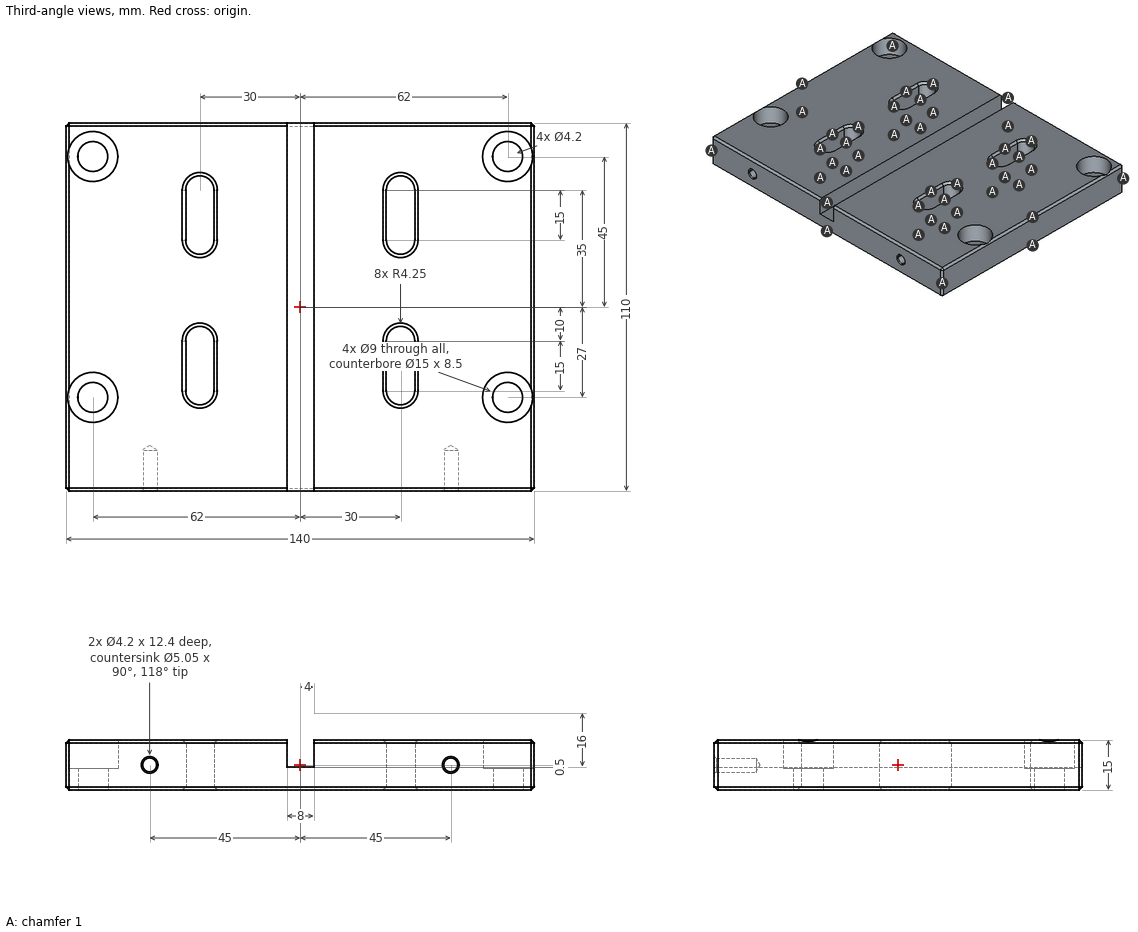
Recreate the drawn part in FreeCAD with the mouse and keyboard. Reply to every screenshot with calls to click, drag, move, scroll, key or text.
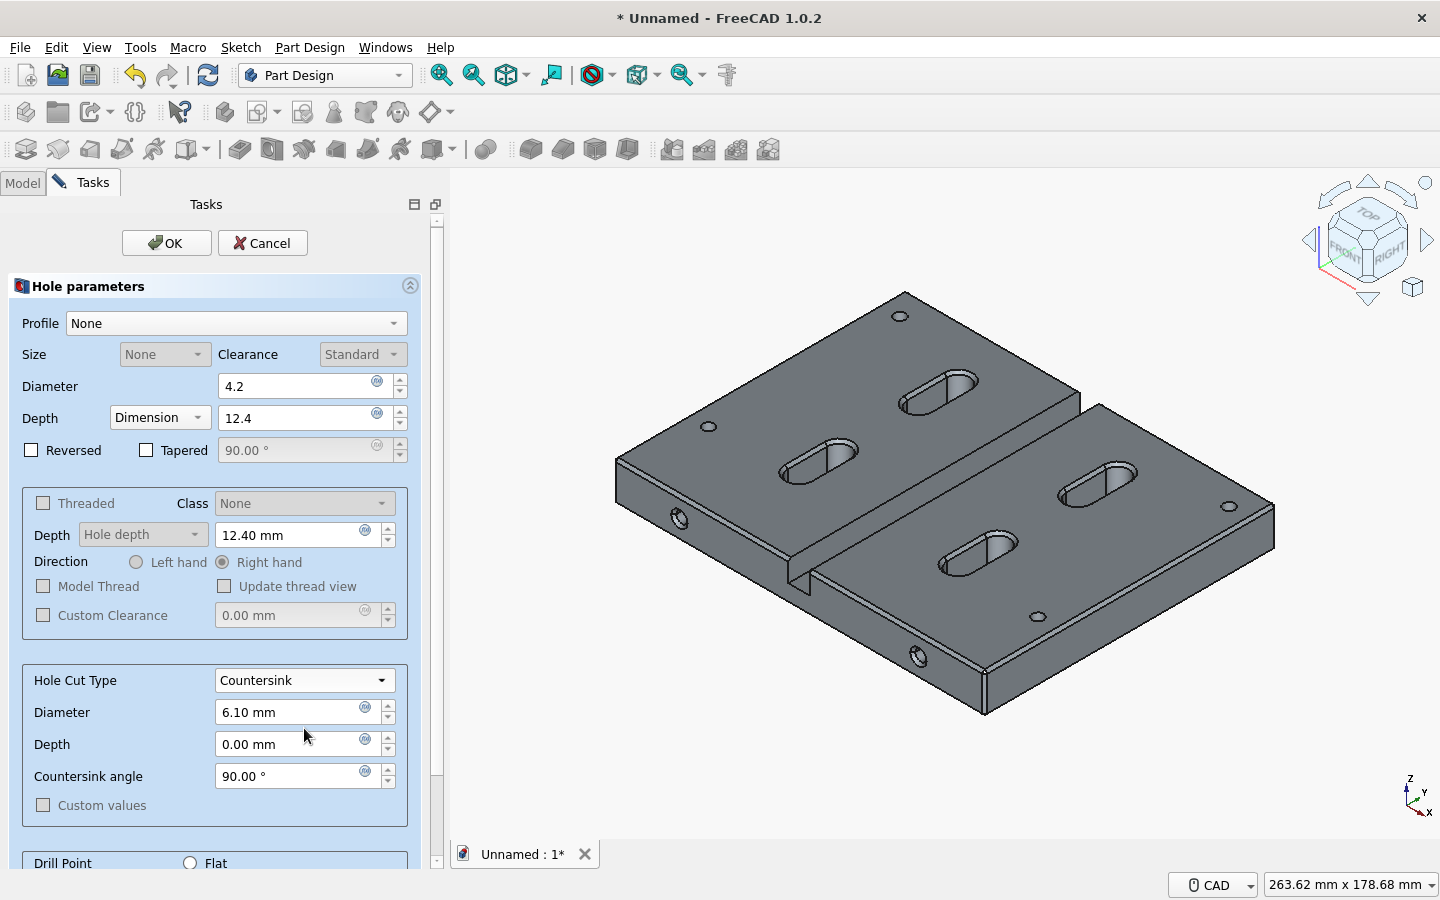
triple_click(298, 712)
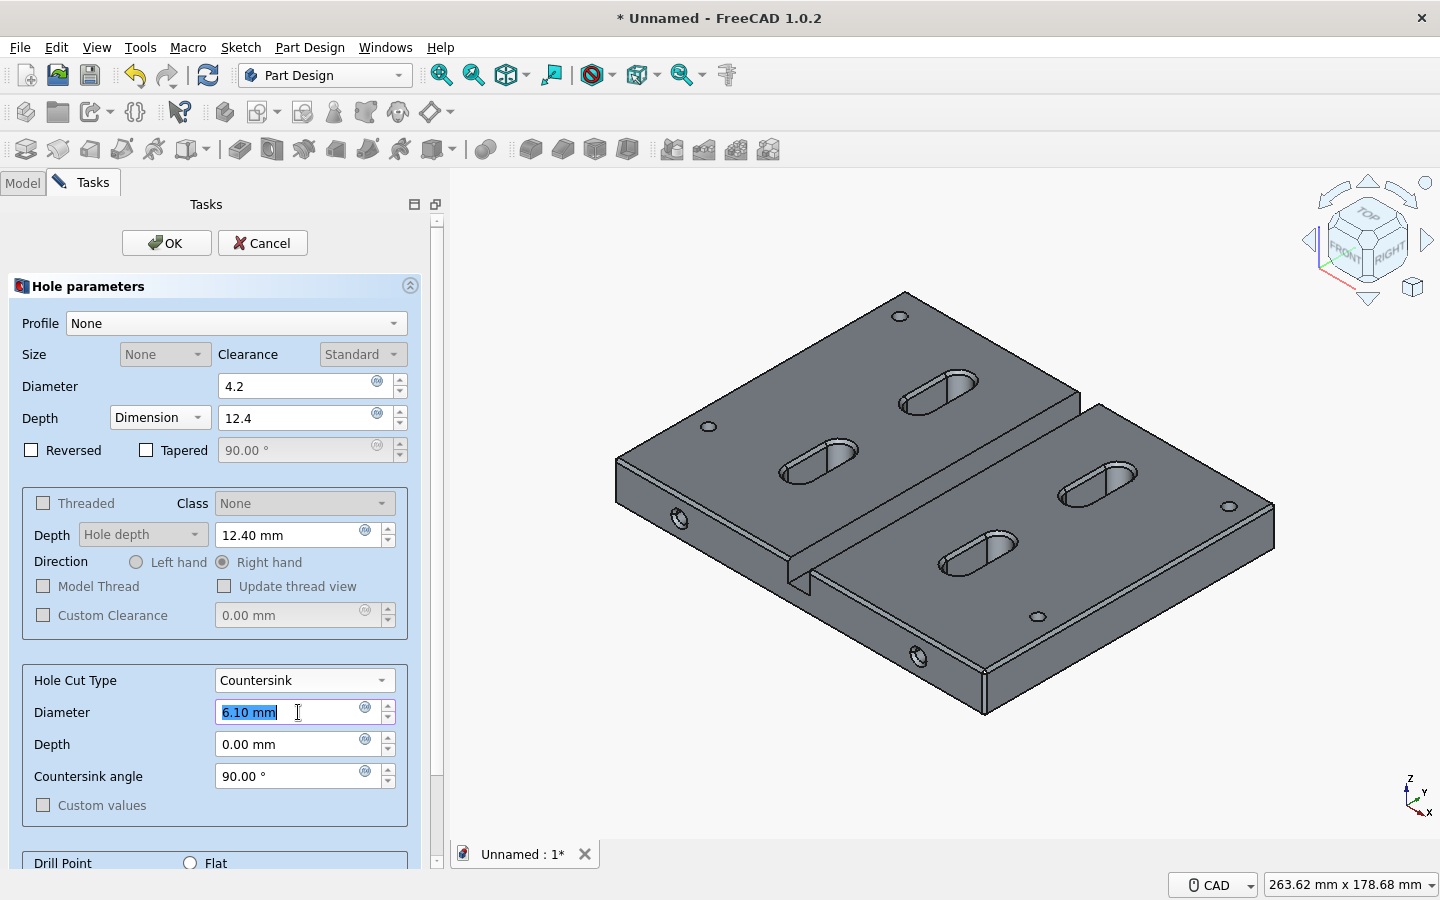
text(5.05)
key(Tab)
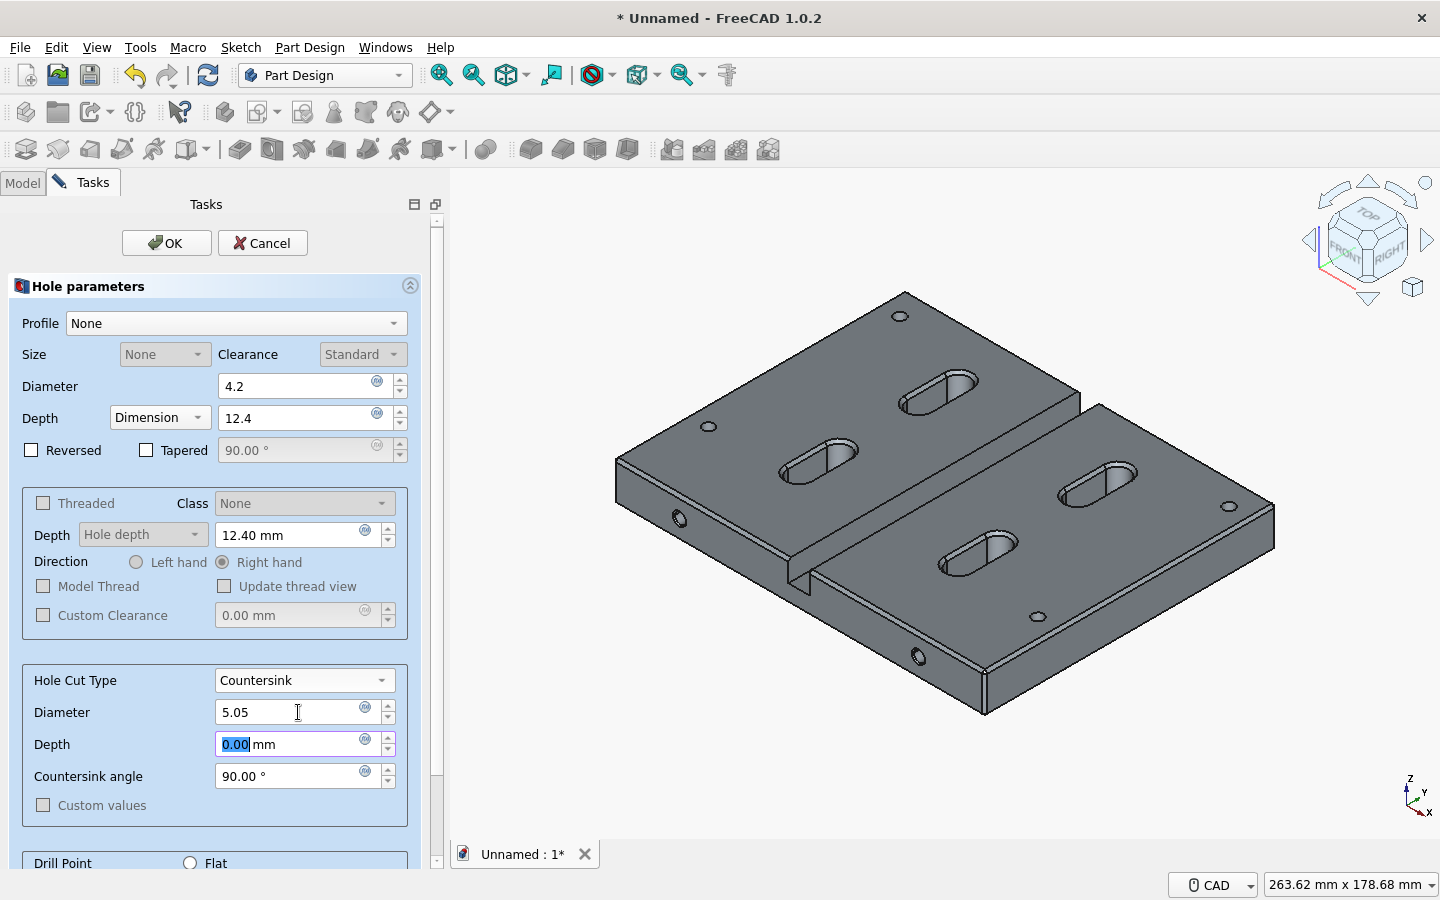
click(167, 243)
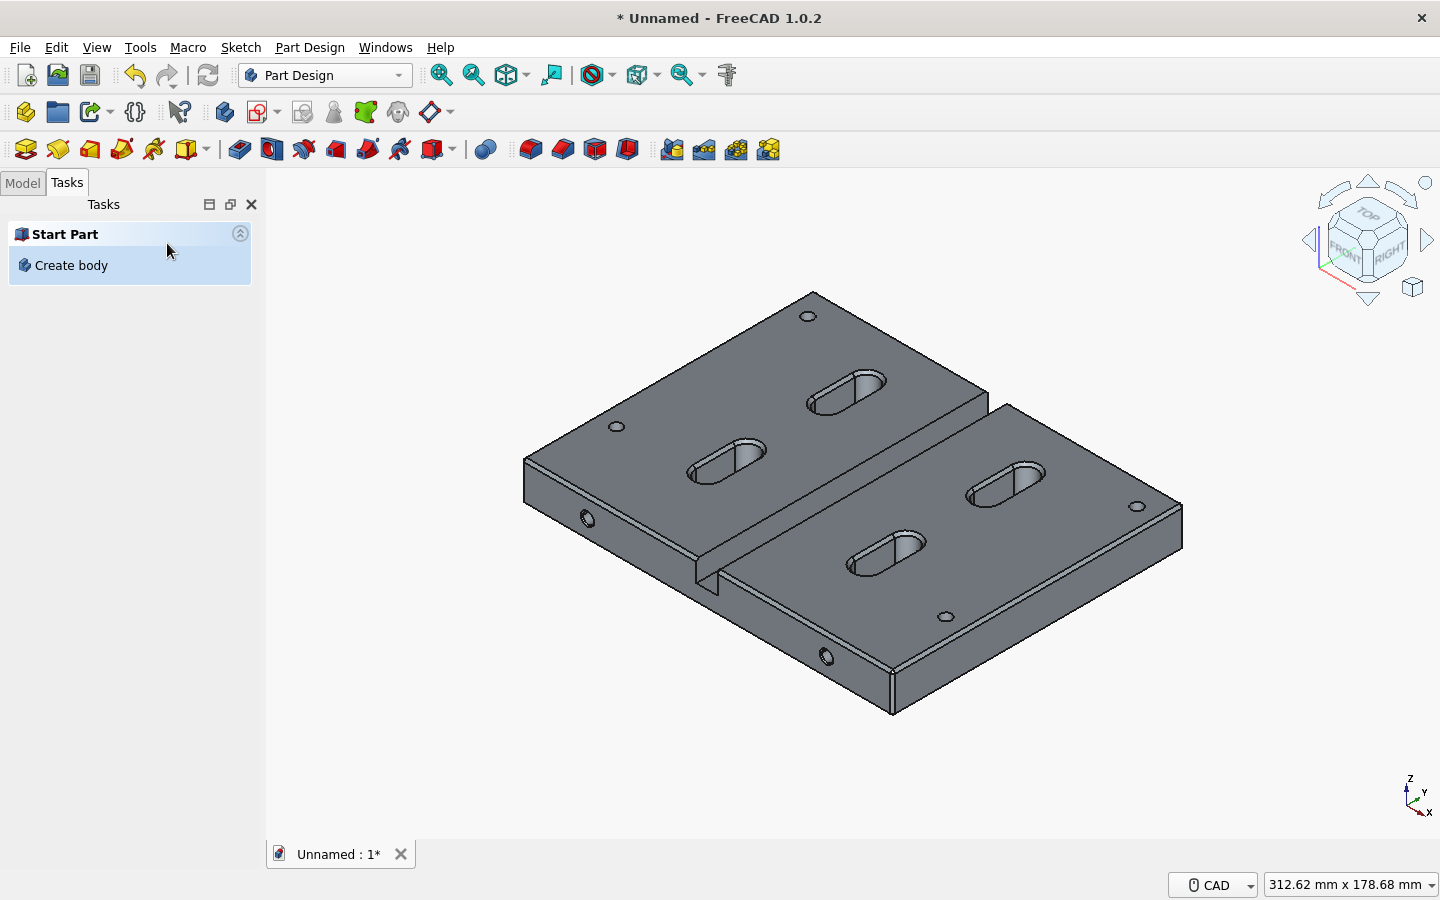
click(1040, 540)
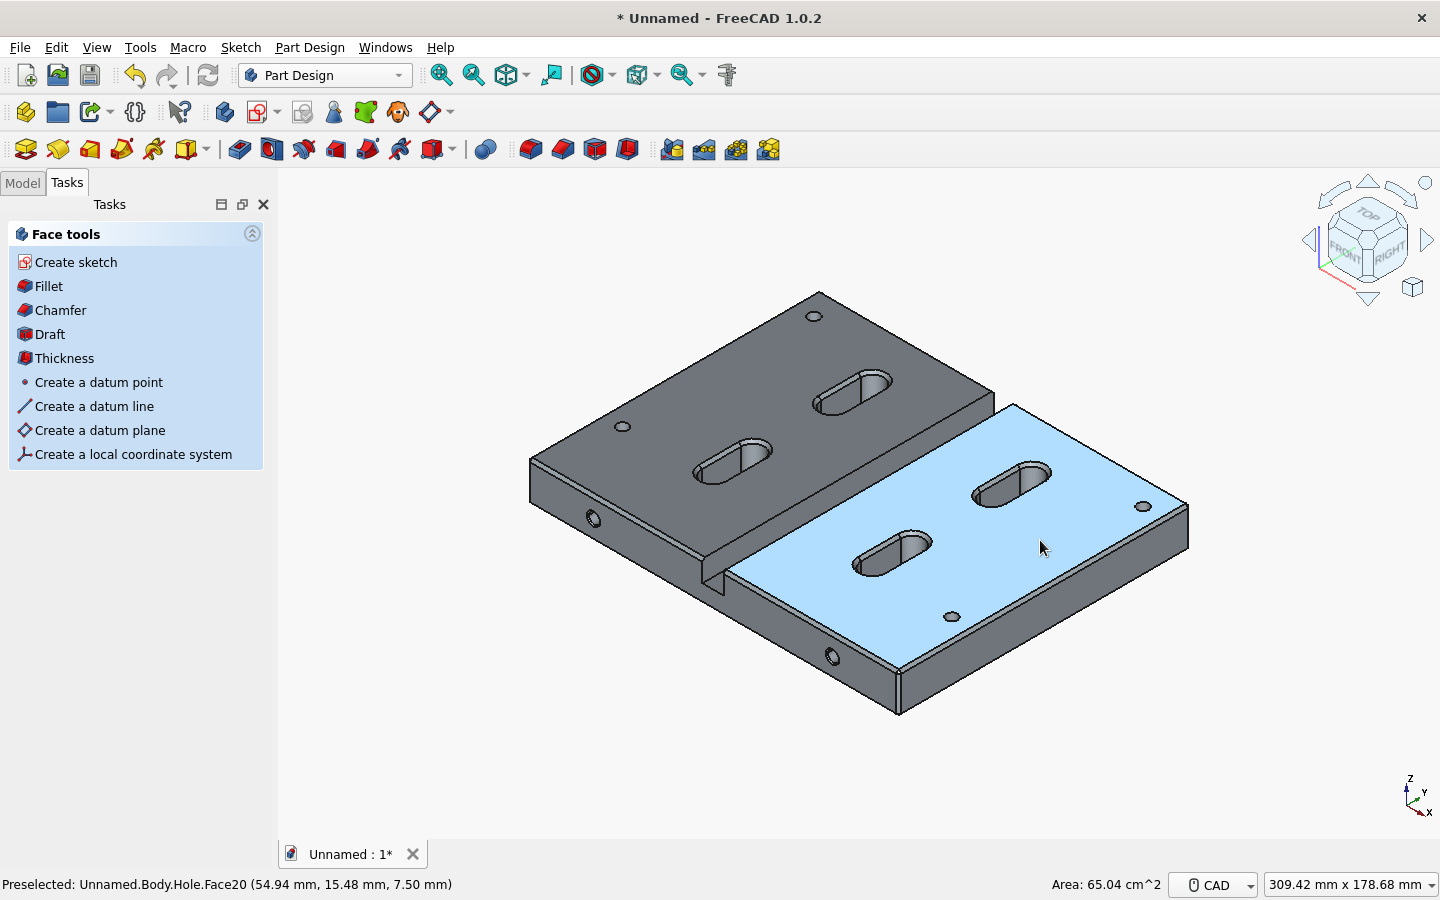
click(258, 112)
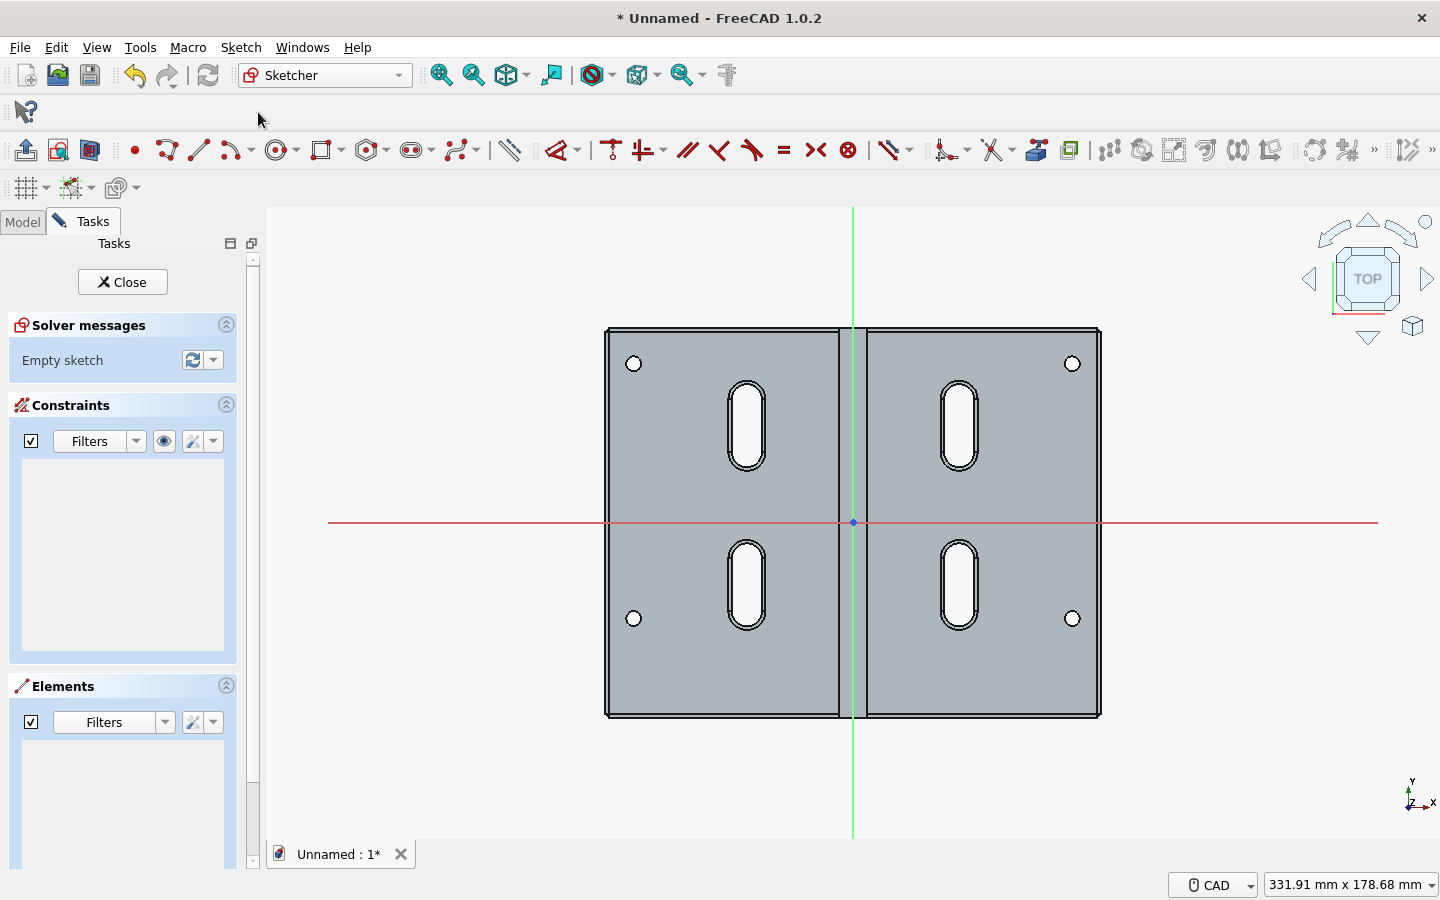
scroll(992, 426, up, 2)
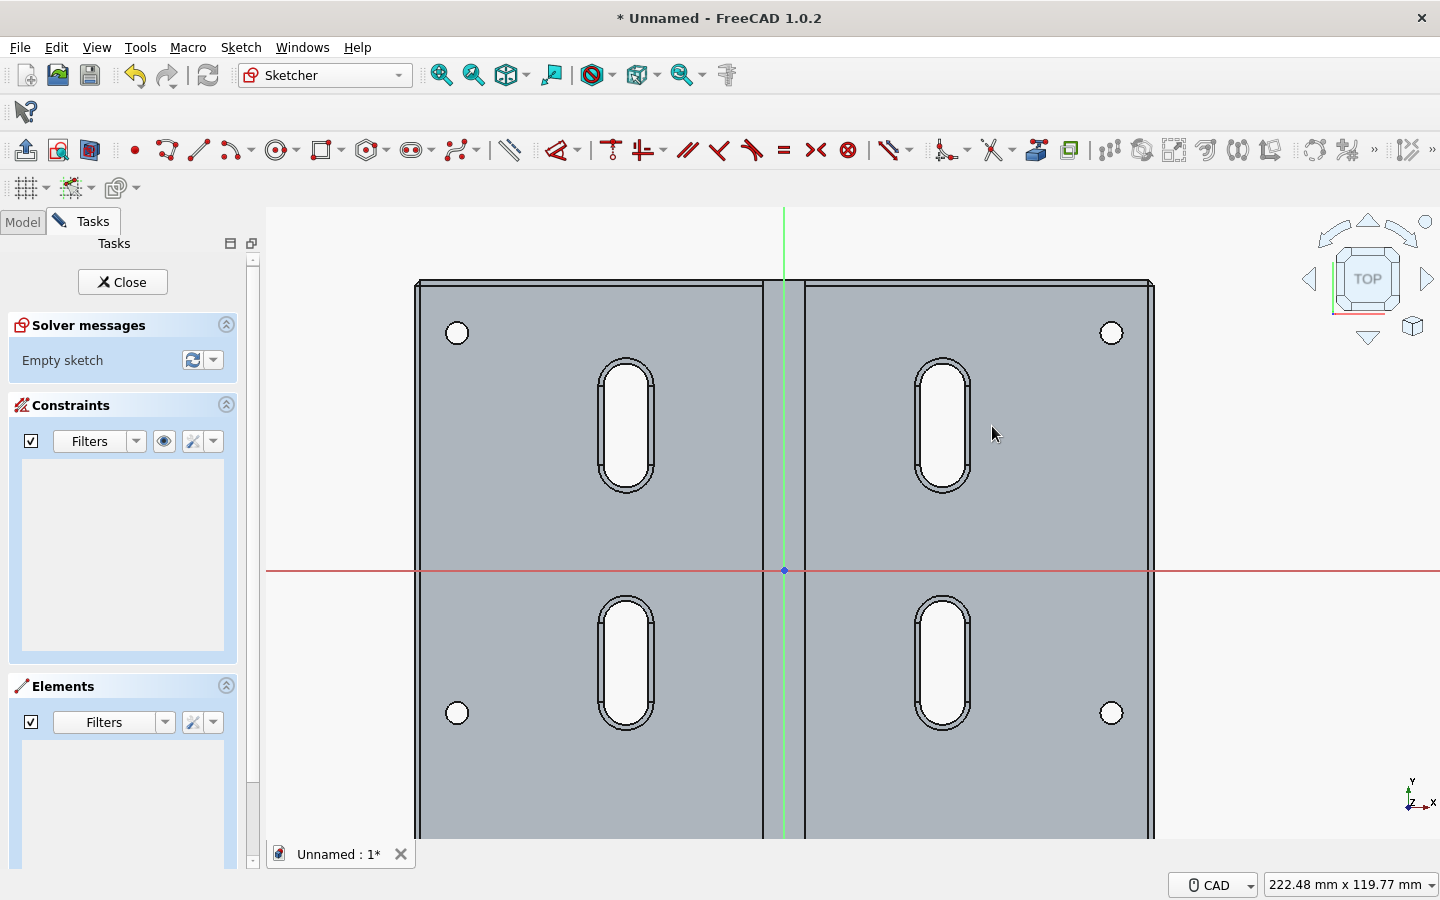
key(g)
key(c)